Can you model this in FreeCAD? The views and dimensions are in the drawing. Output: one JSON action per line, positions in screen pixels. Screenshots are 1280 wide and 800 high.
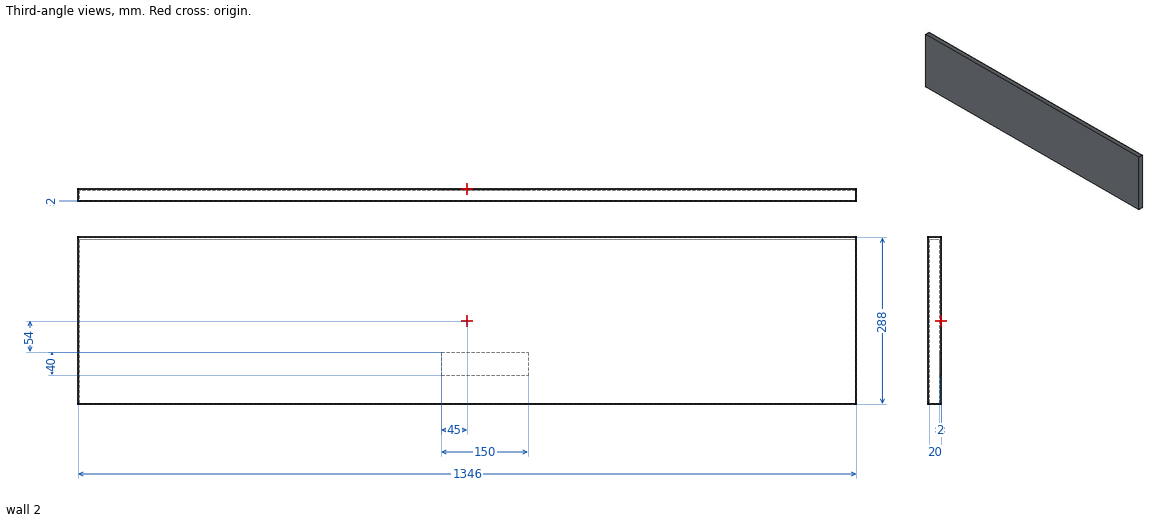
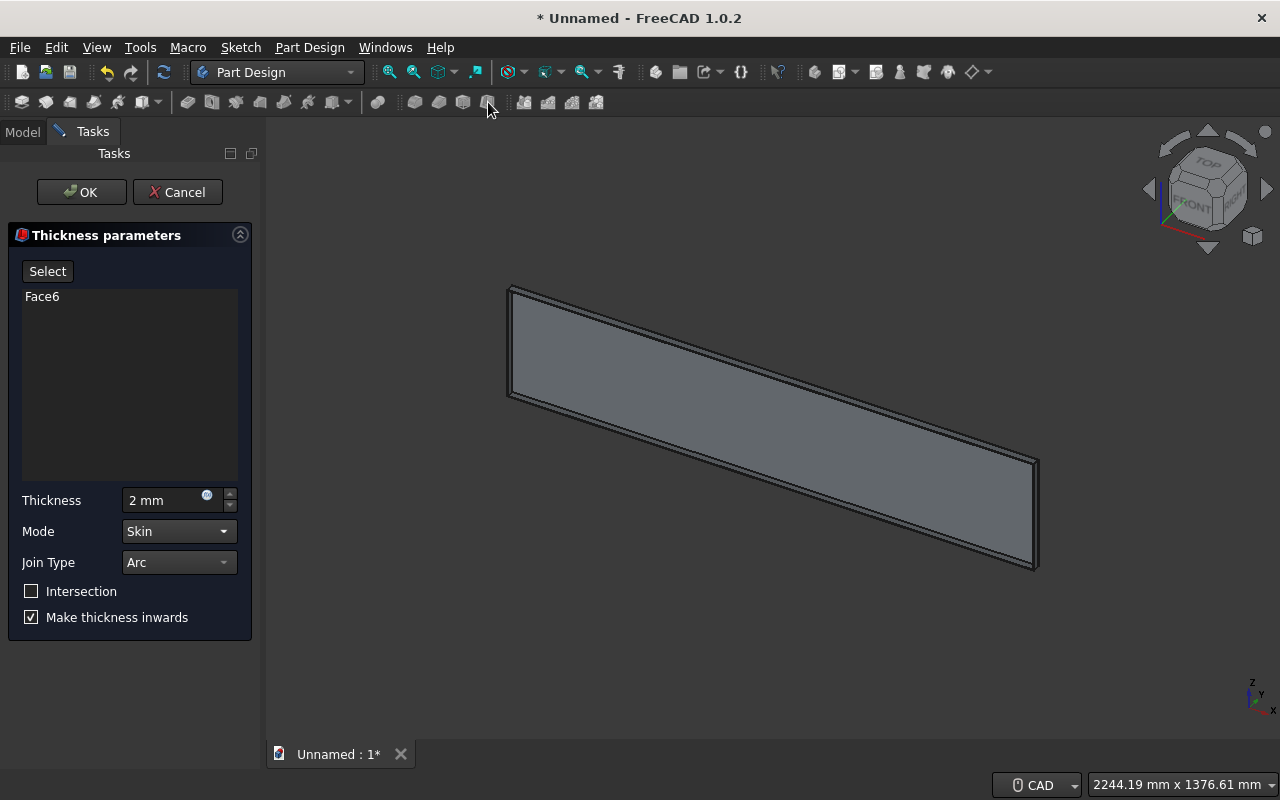
{"action": "left_click", "coordinate": [180, 562]}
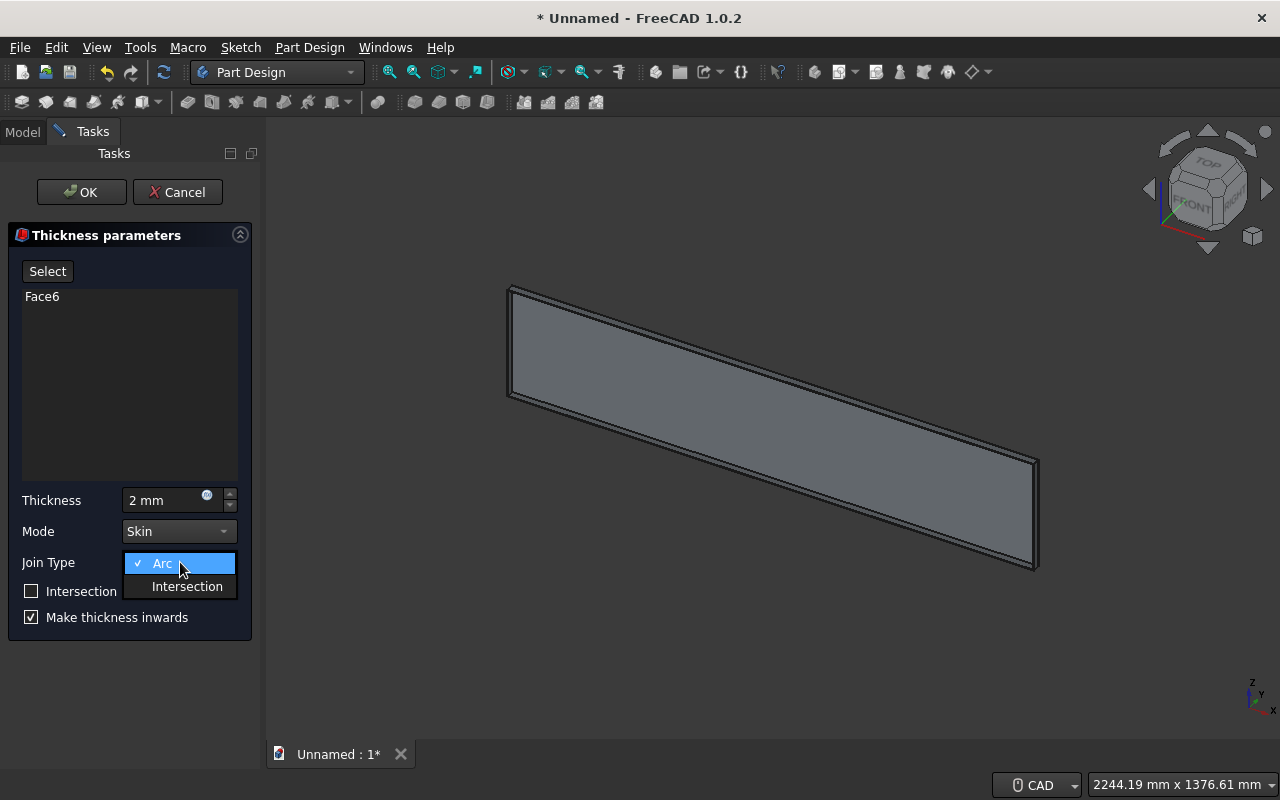
{"action": "left_click", "coordinate": [179, 586]}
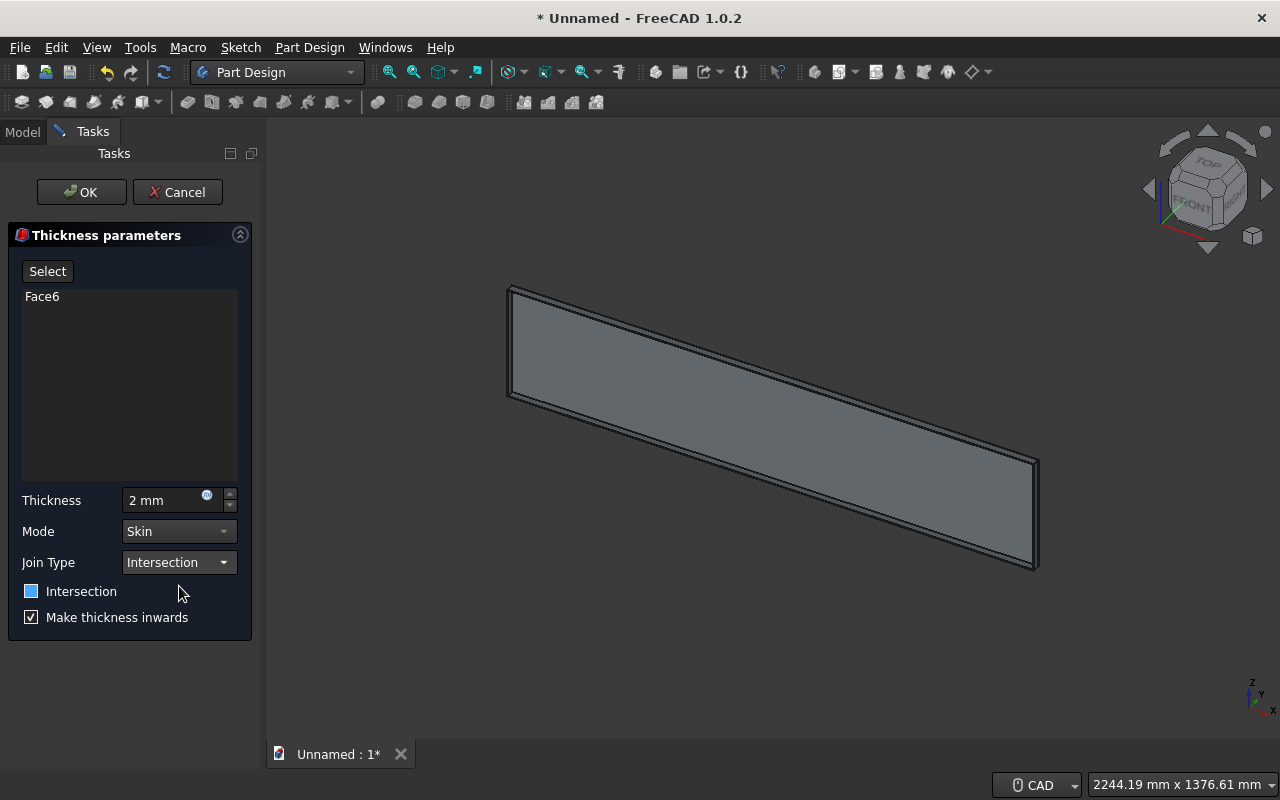
{"action": "left_click", "coordinate": [82, 192]}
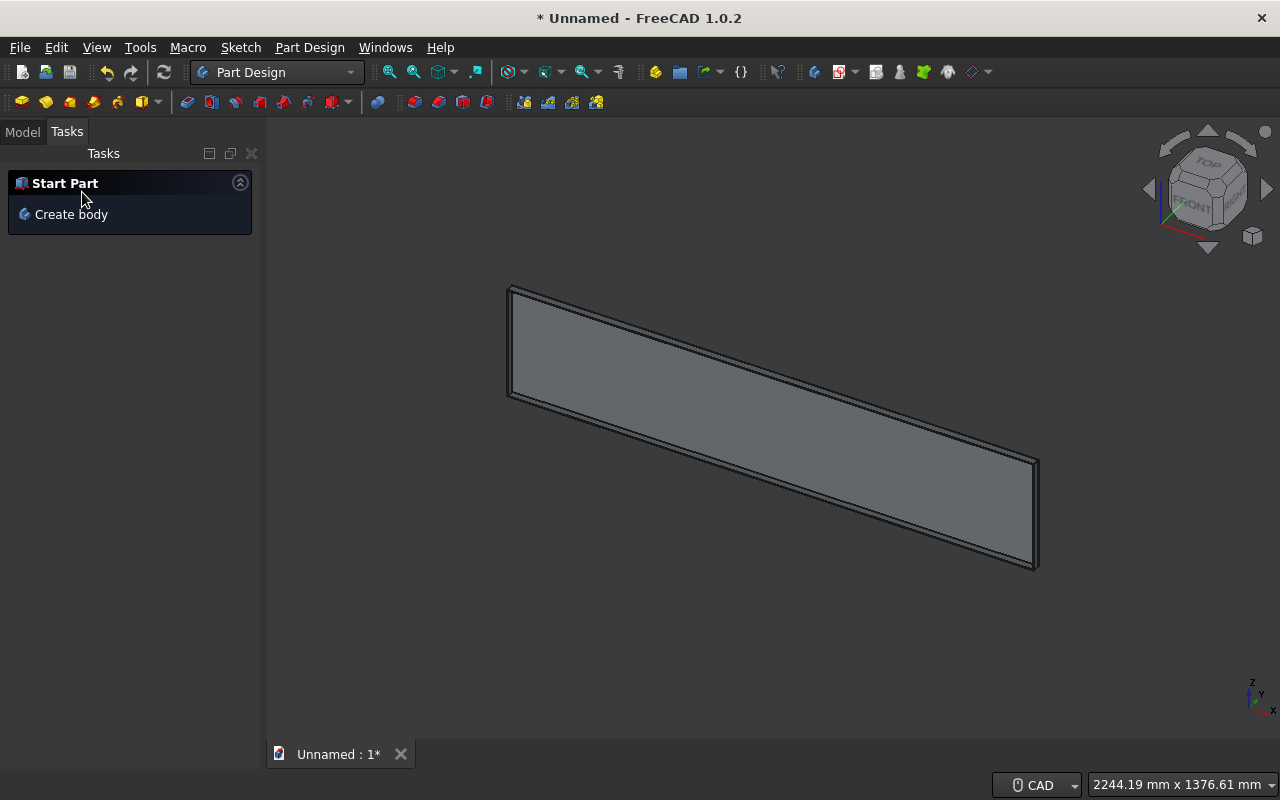
{"action": "scroll", "coordinate": [1034, 499], "scroll_direction": "up", "scroll_amount": 15}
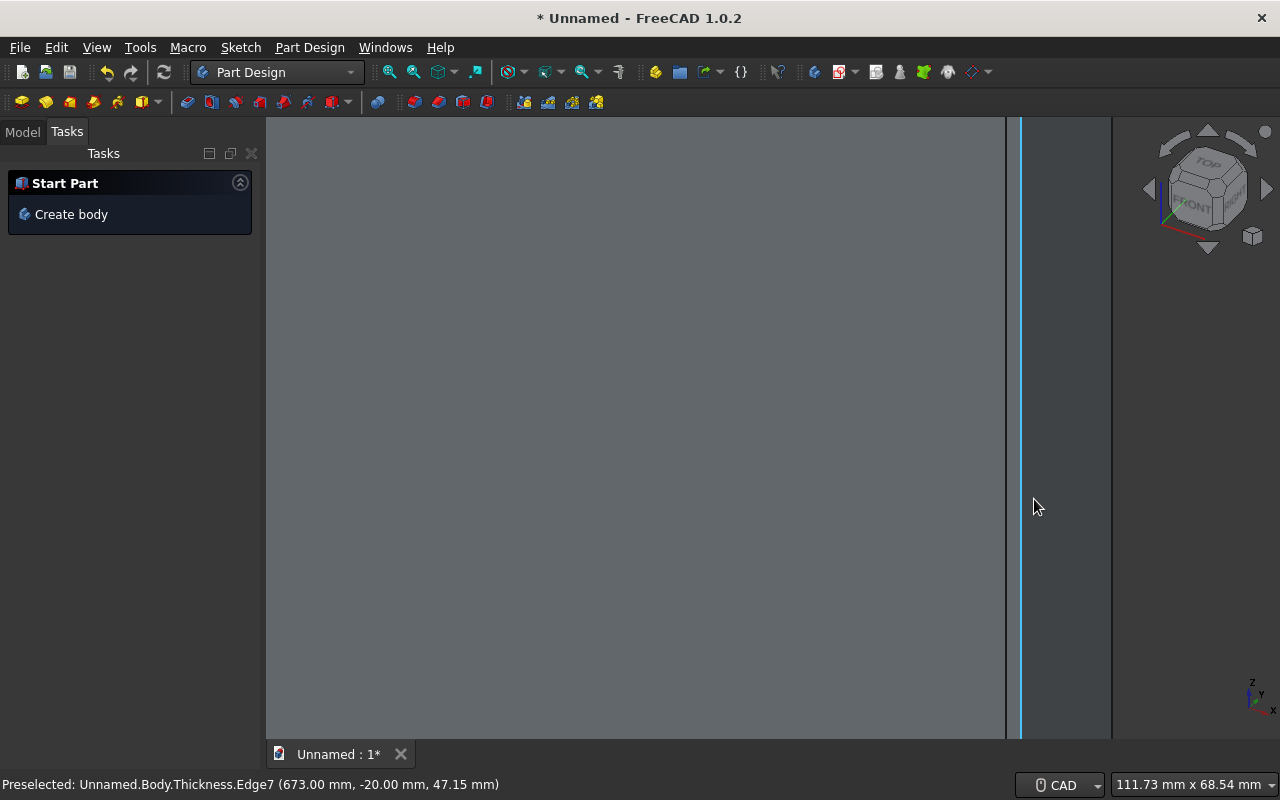
{"action": "left_click", "coordinate": [1011, 497]}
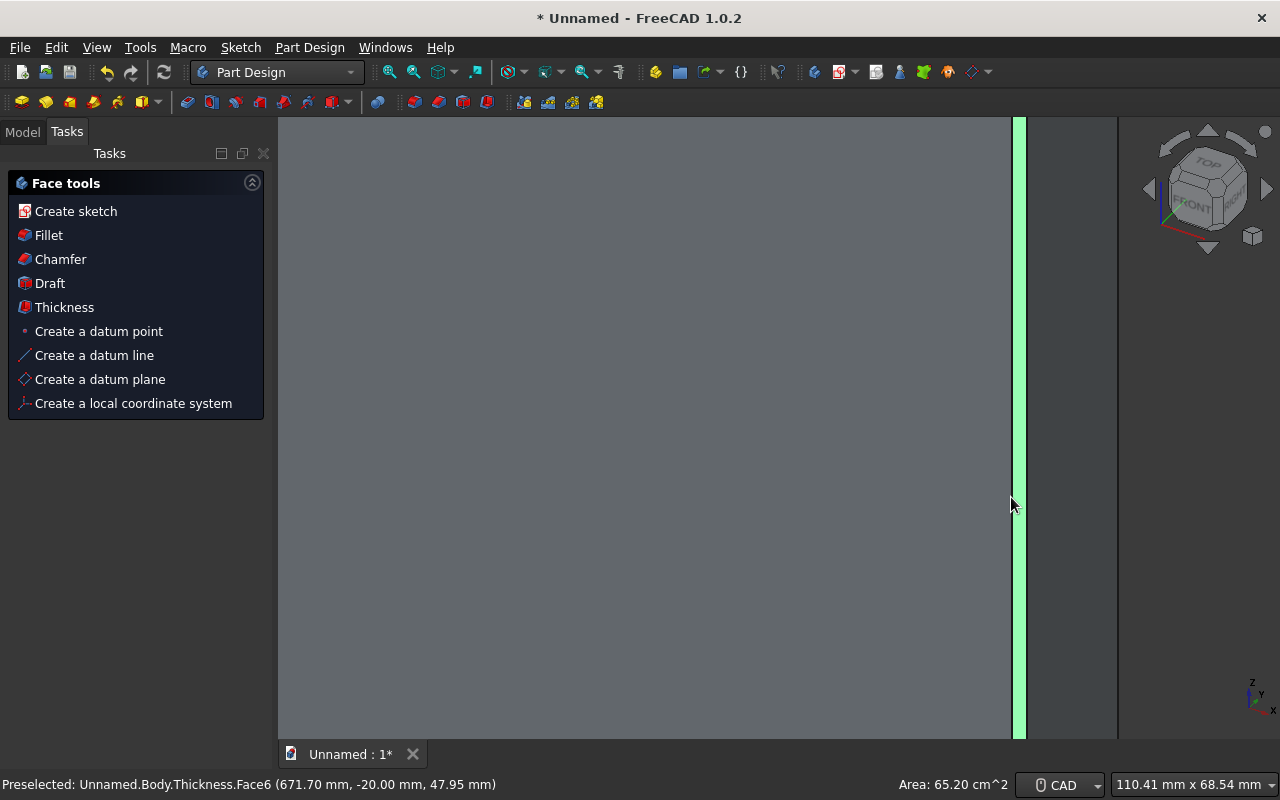
{"action": "left_click", "coordinate": [840, 72]}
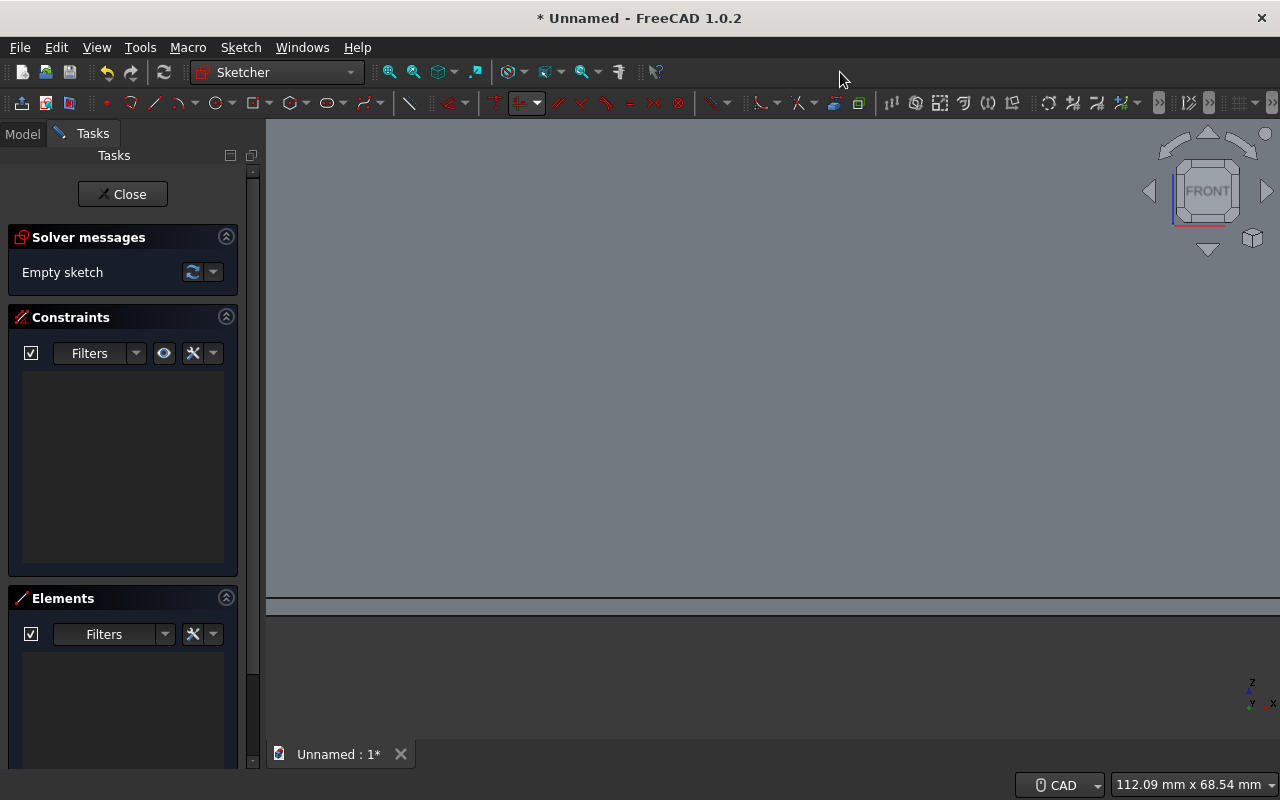
{"action": "scroll", "coordinate": [947, 487], "scroll_direction": "down", "scroll_amount": 15}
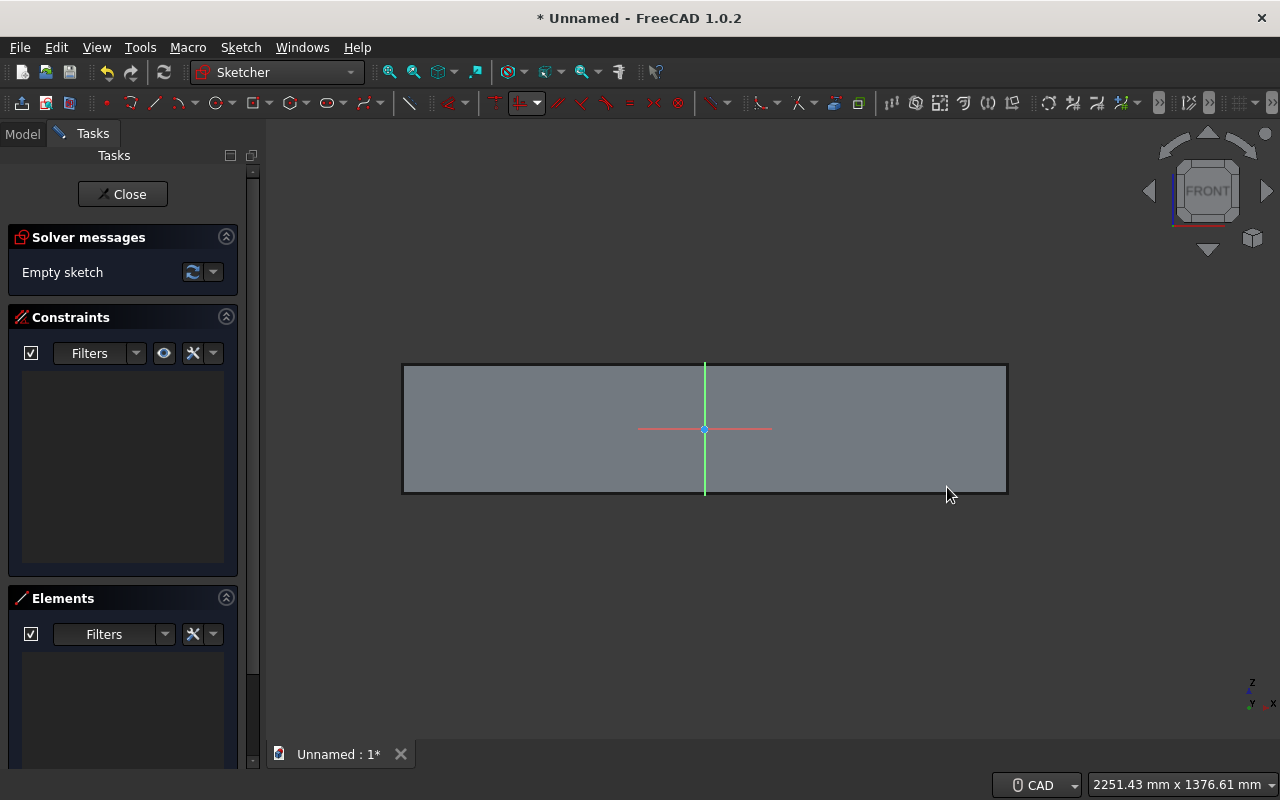
{"action": "key", "text": "g v"}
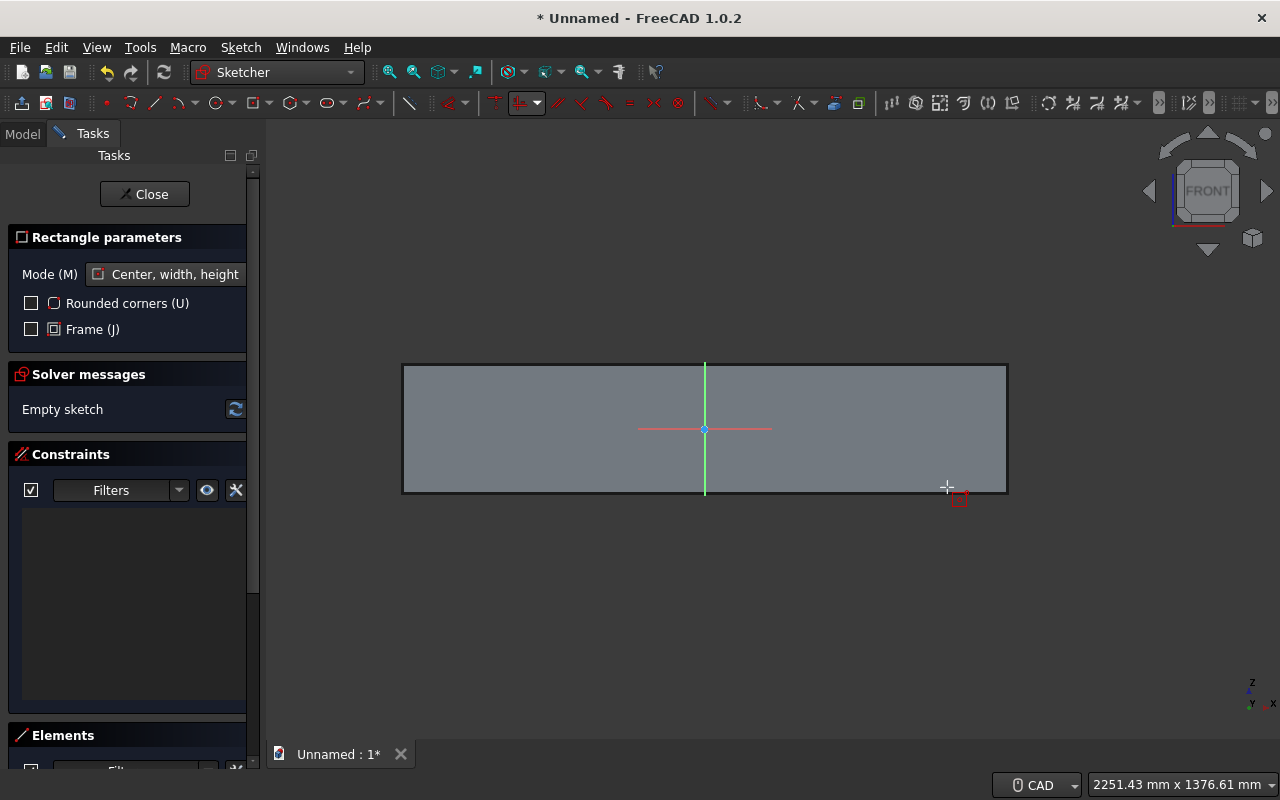
{"action": "left_click", "coordinate": [705, 429]}
{"action": "left_click", "coordinate": [1008, 364]}
{"action": "key", "text": "Escape"}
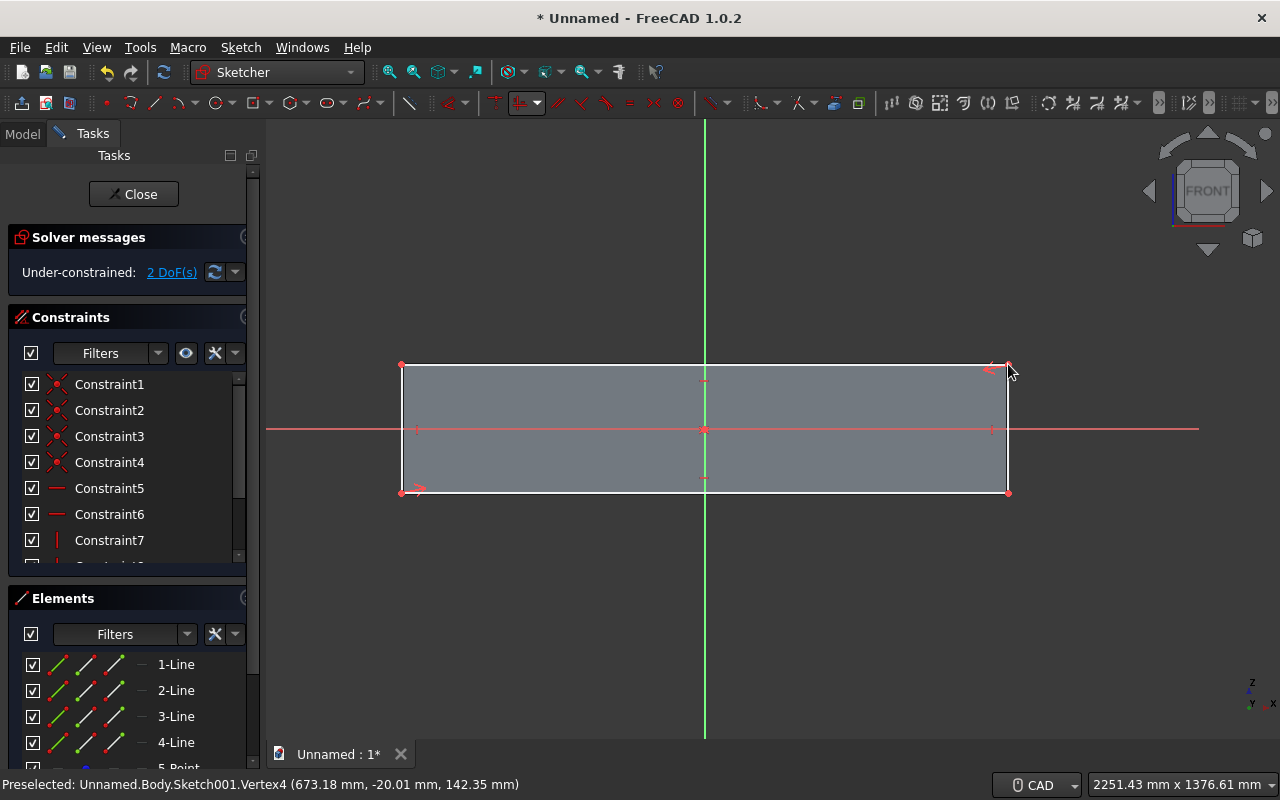
{"action": "left_click", "coordinate": [448, 104]}